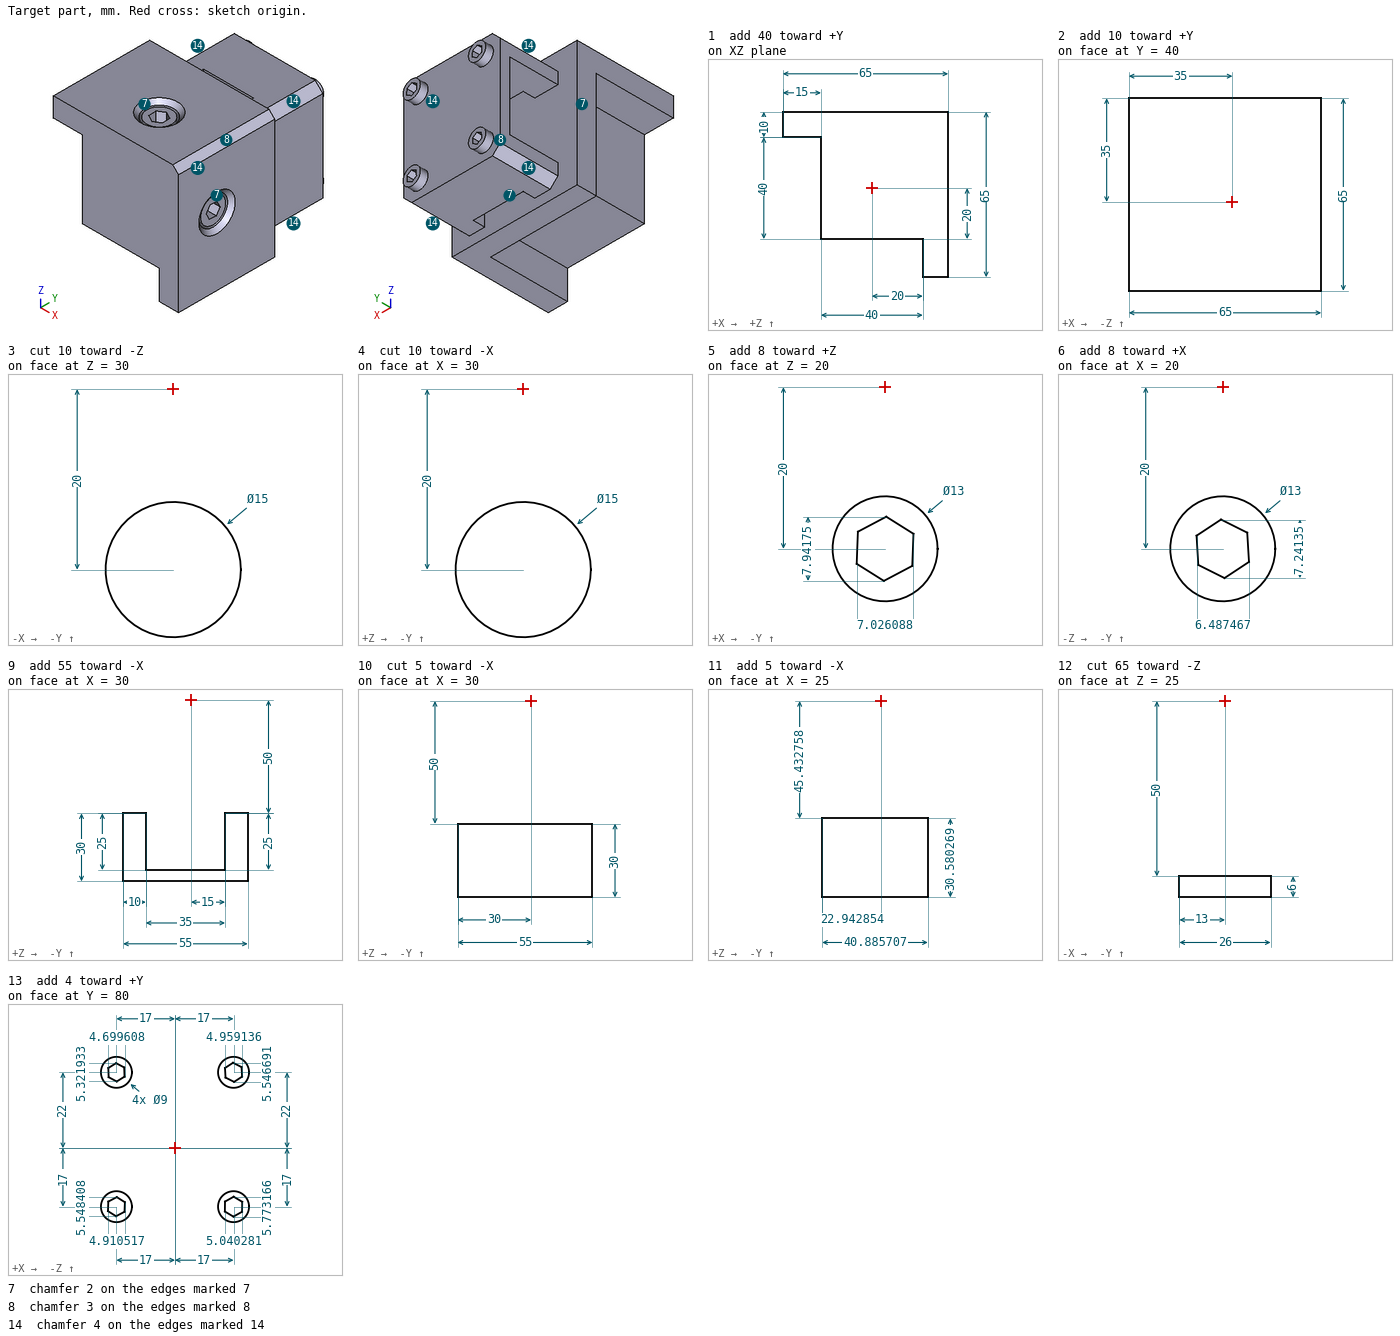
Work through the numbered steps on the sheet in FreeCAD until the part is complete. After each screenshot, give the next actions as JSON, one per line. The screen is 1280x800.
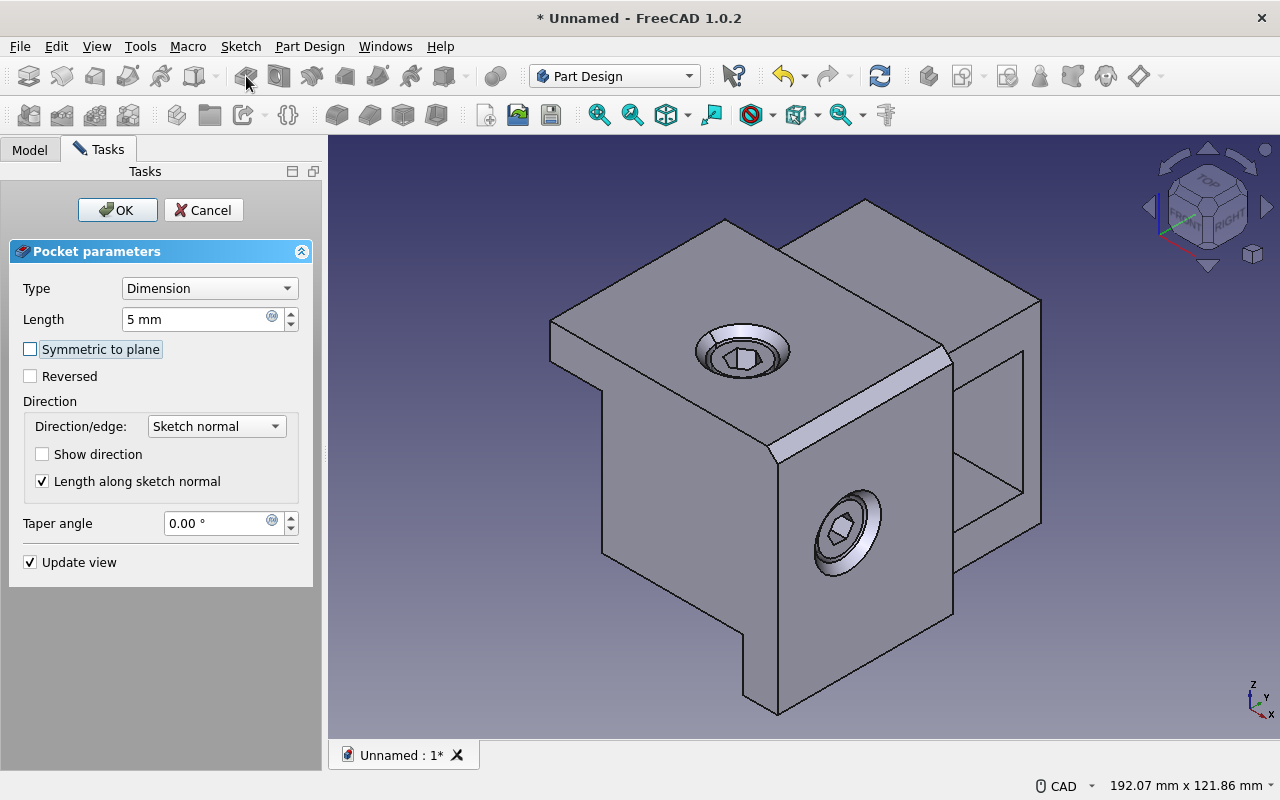
{"action": "left_click", "coordinate": [118, 210]}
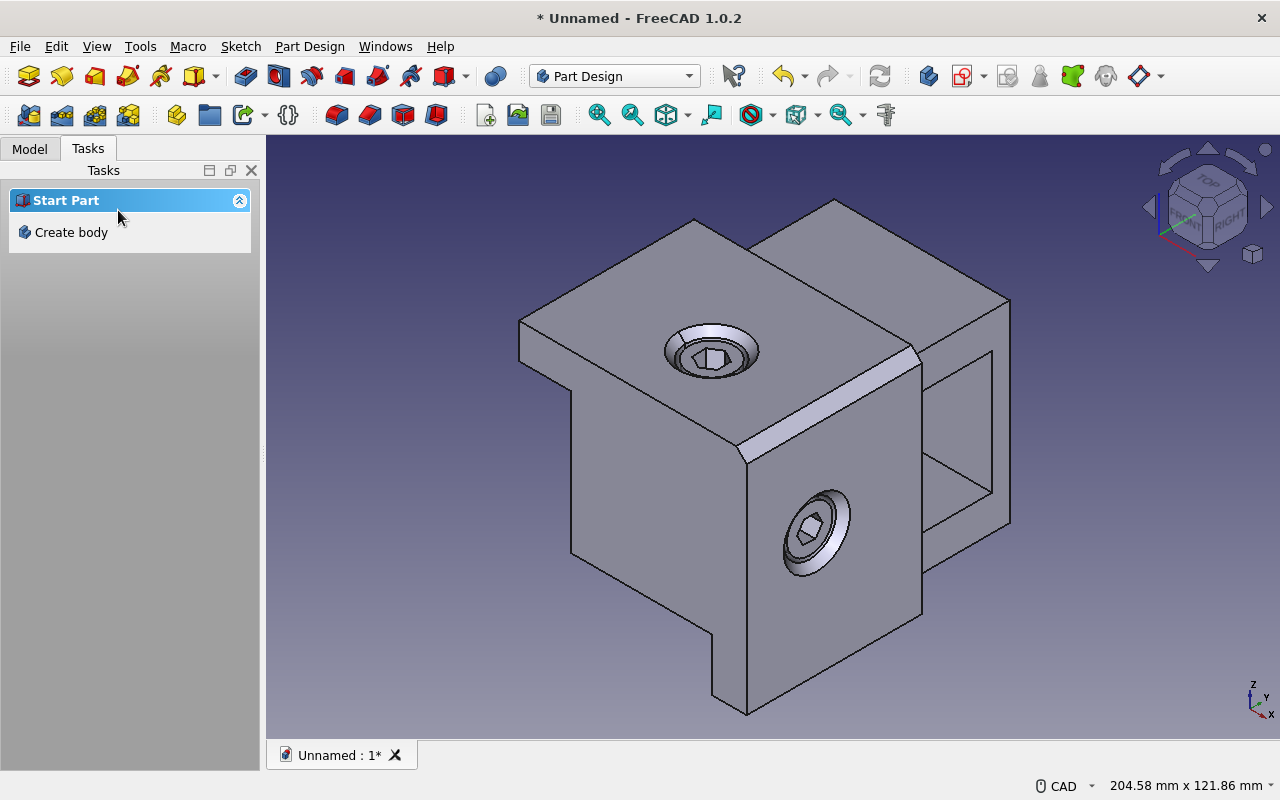
{"action": "left_click", "coordinate": [987, 328]}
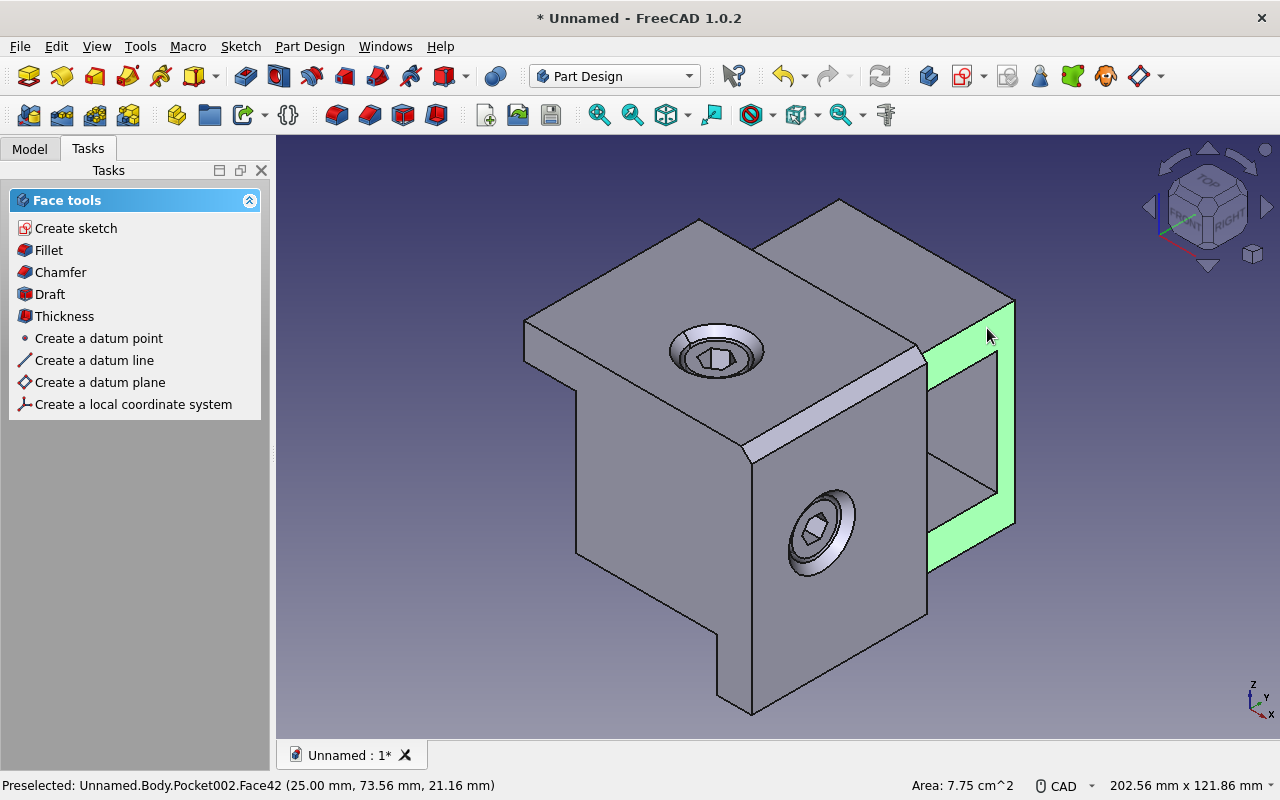
{"action": "left_click", "coordinate": [962, 76]}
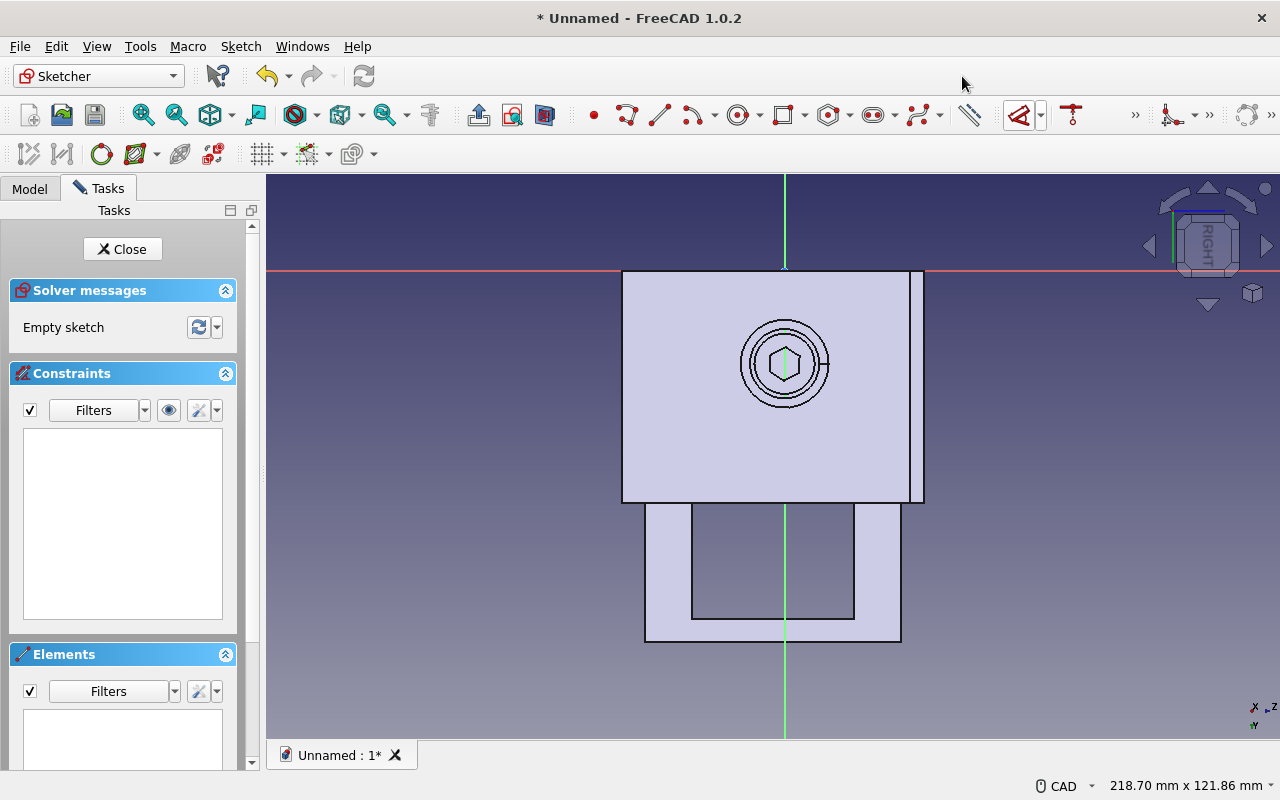
{"action": "left_click", "coordinate": [545, 116]}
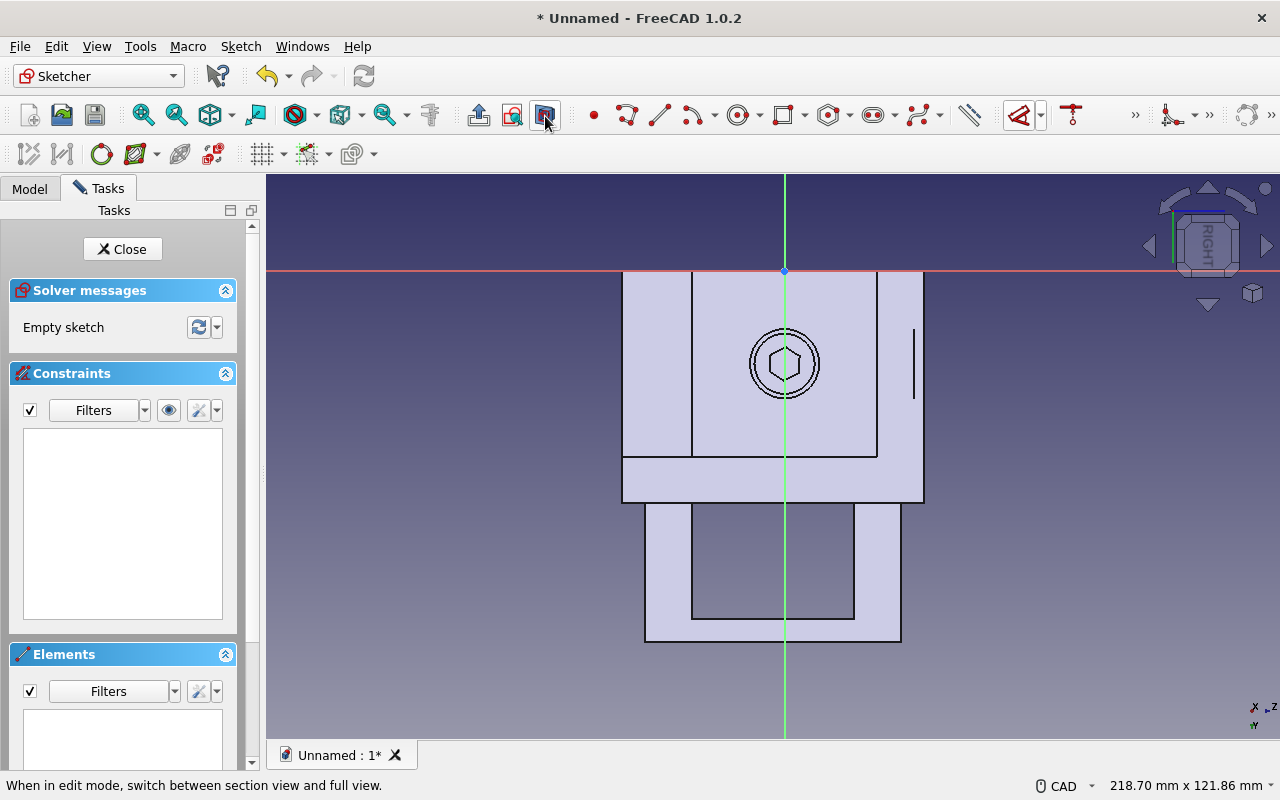
{"action": "left_click", "coordinate": [782, 116]}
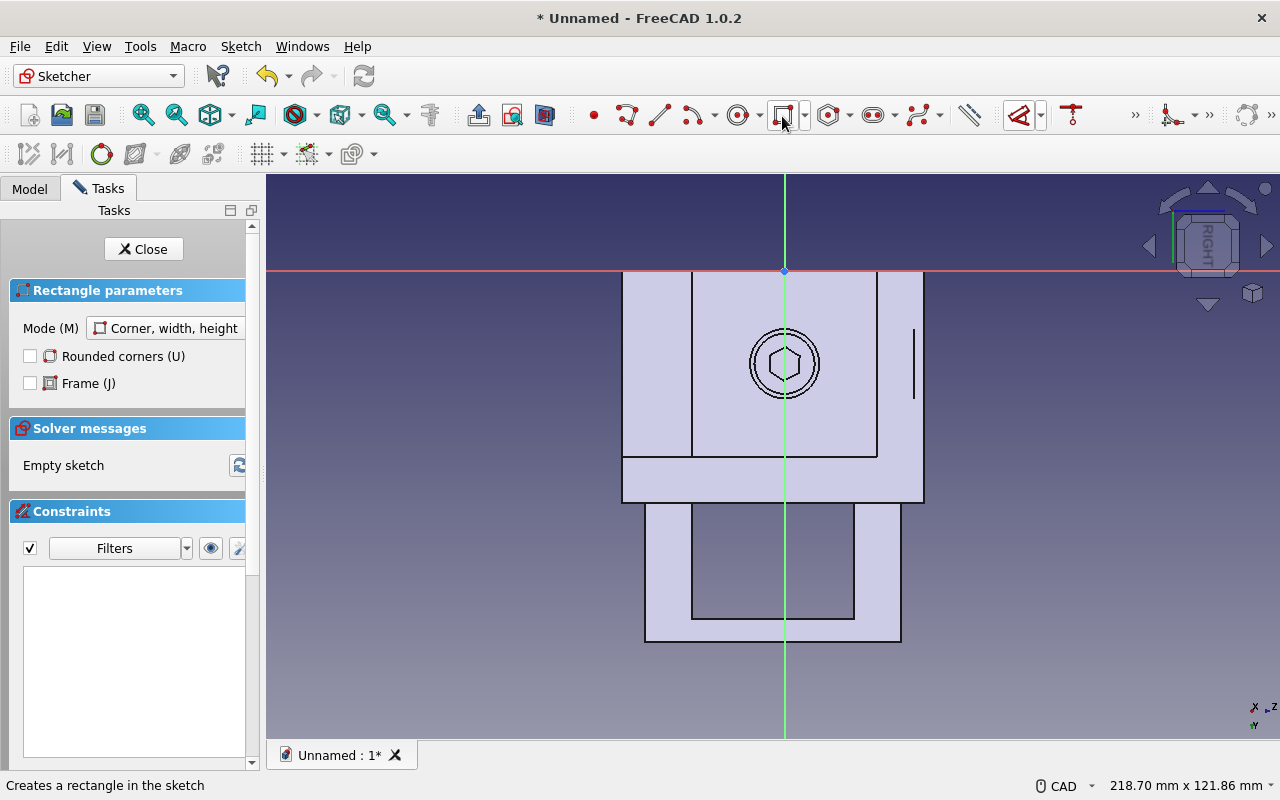
{"action": "left_click", "coordinate": [678, 482]}
{"action": "mouse_move", "coordinate": [868, 623]}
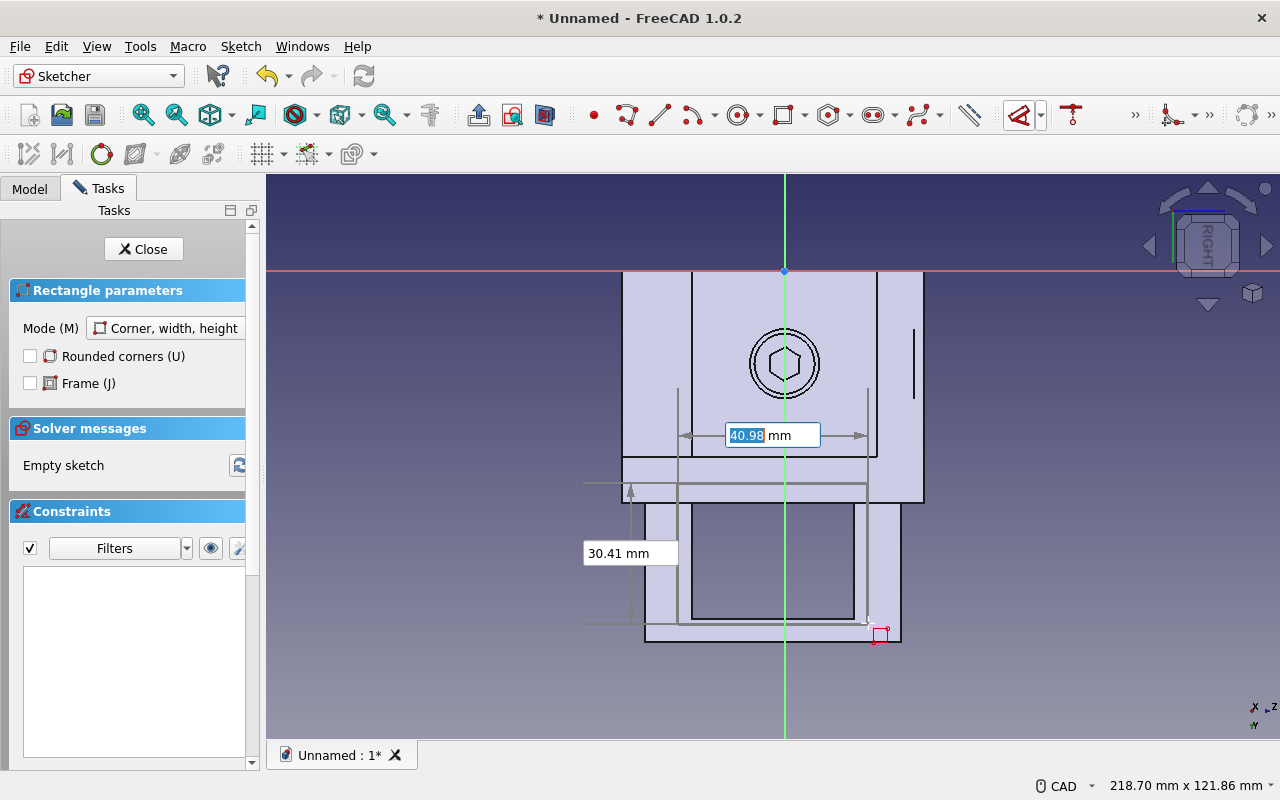
{"action": "type", "text": "40.885707"}
{"action": "key", "text": "Tab"}
{"action": "type", "text": "30.580269"}
{"action": "key", "text": "Return"}
{"action": "key", "text": "Escape"}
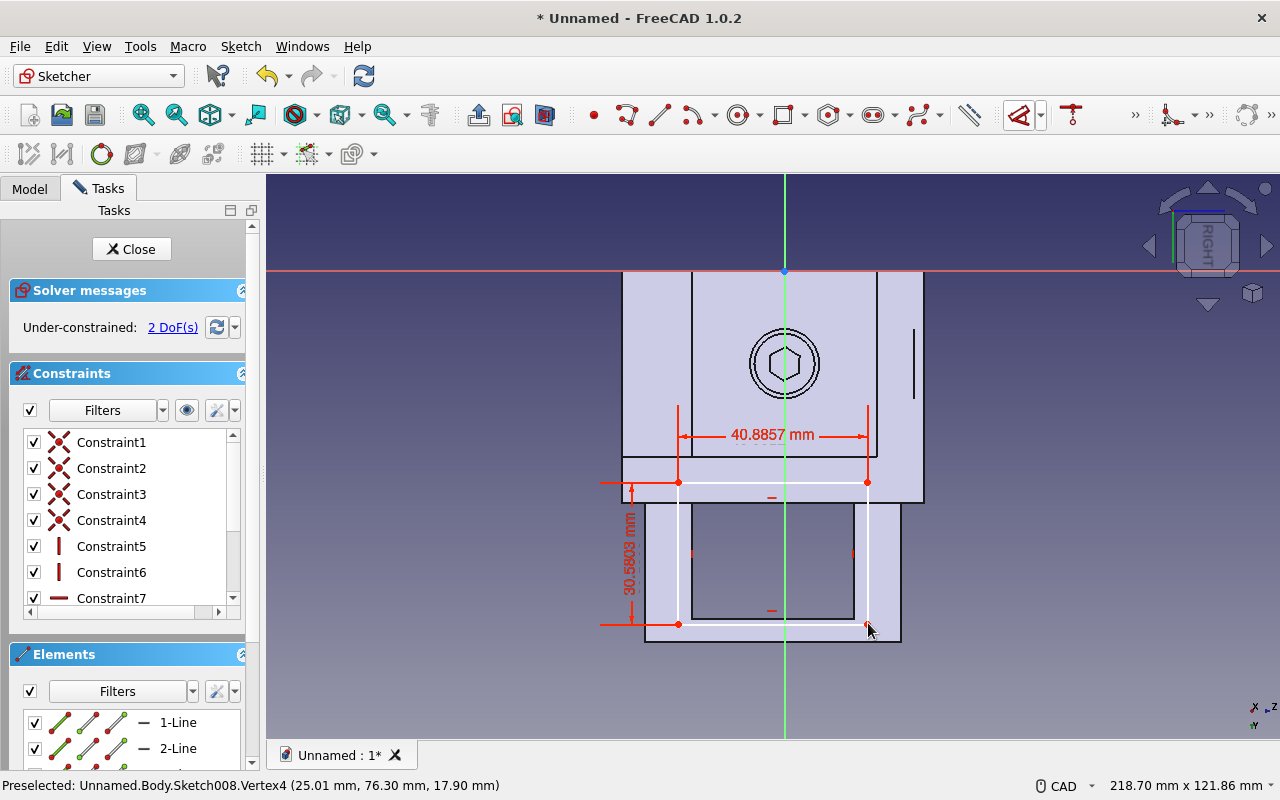
{"action": "left_click", "coordinate": [678, 483]}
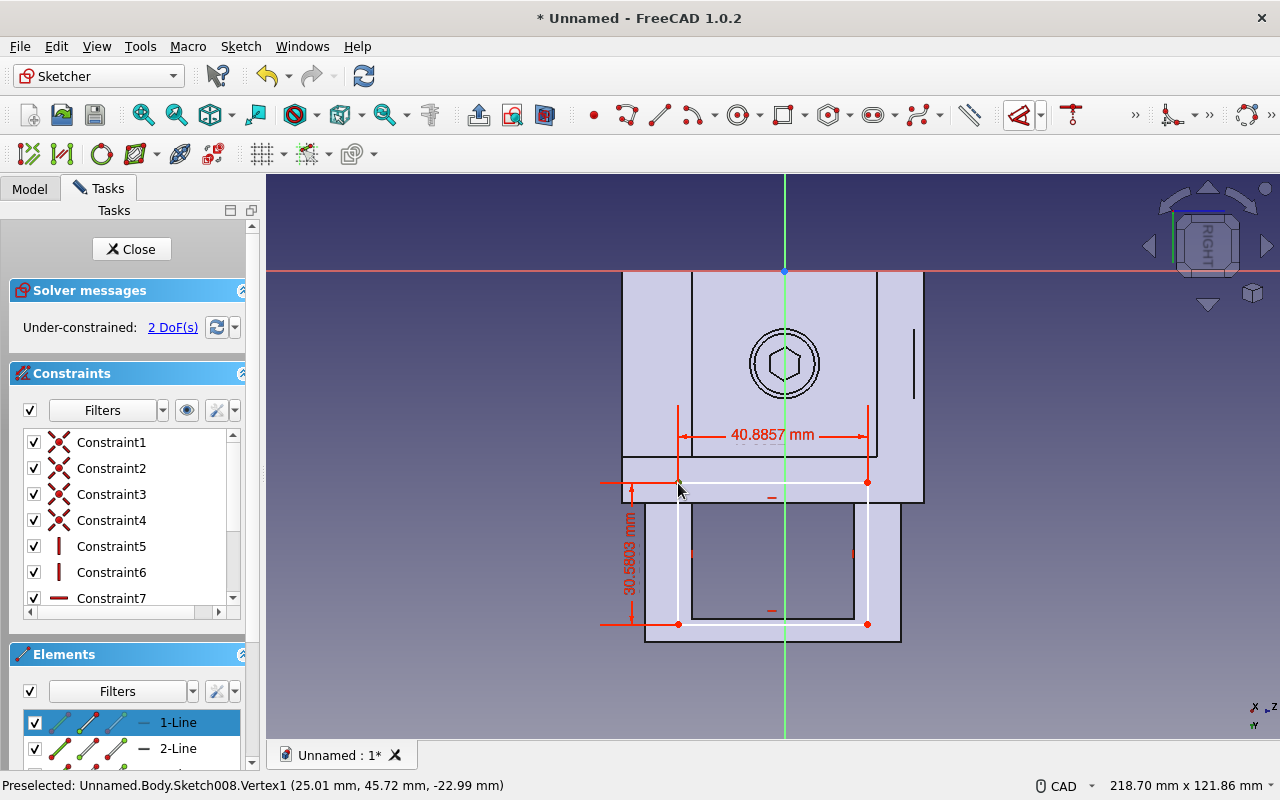
{"action": "left_click", "coordinate": [1040, 116]}